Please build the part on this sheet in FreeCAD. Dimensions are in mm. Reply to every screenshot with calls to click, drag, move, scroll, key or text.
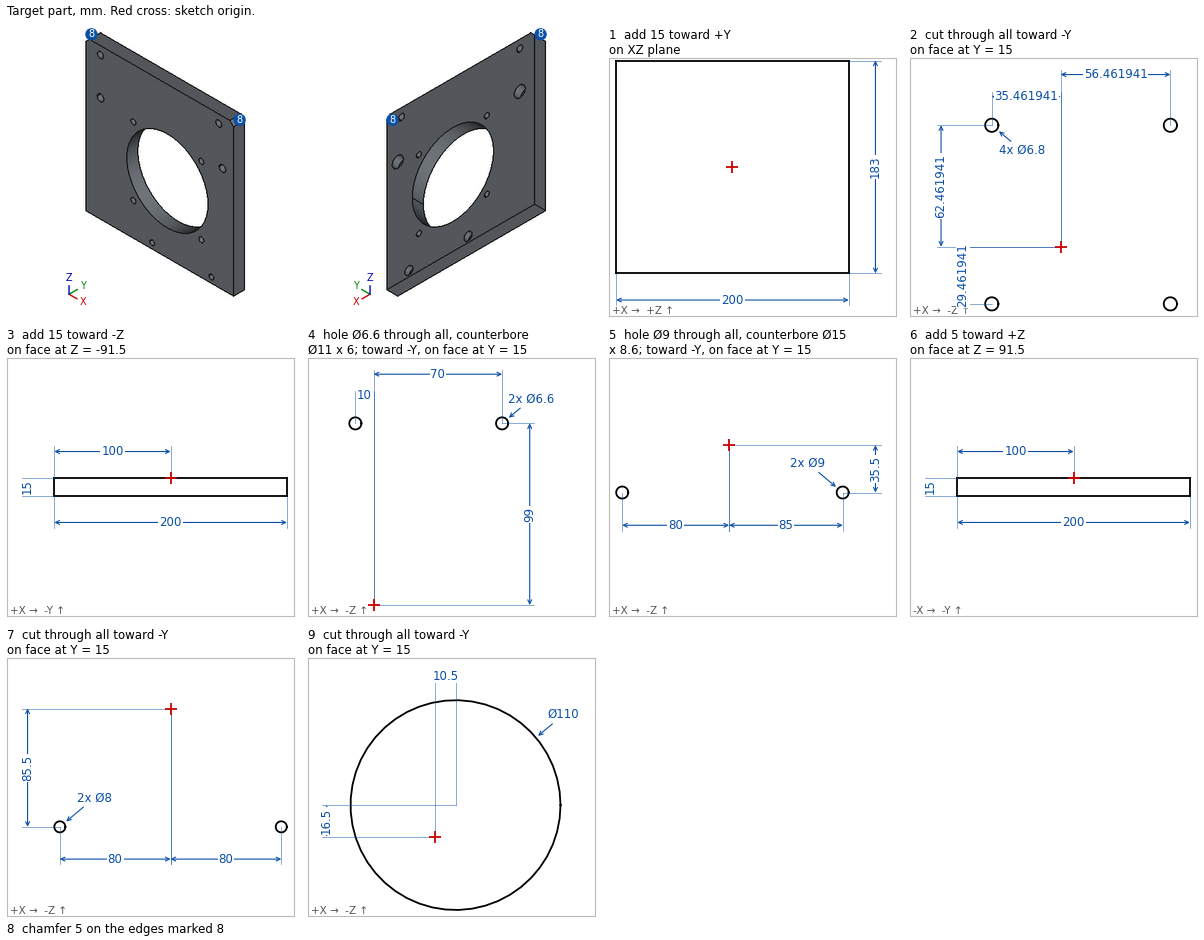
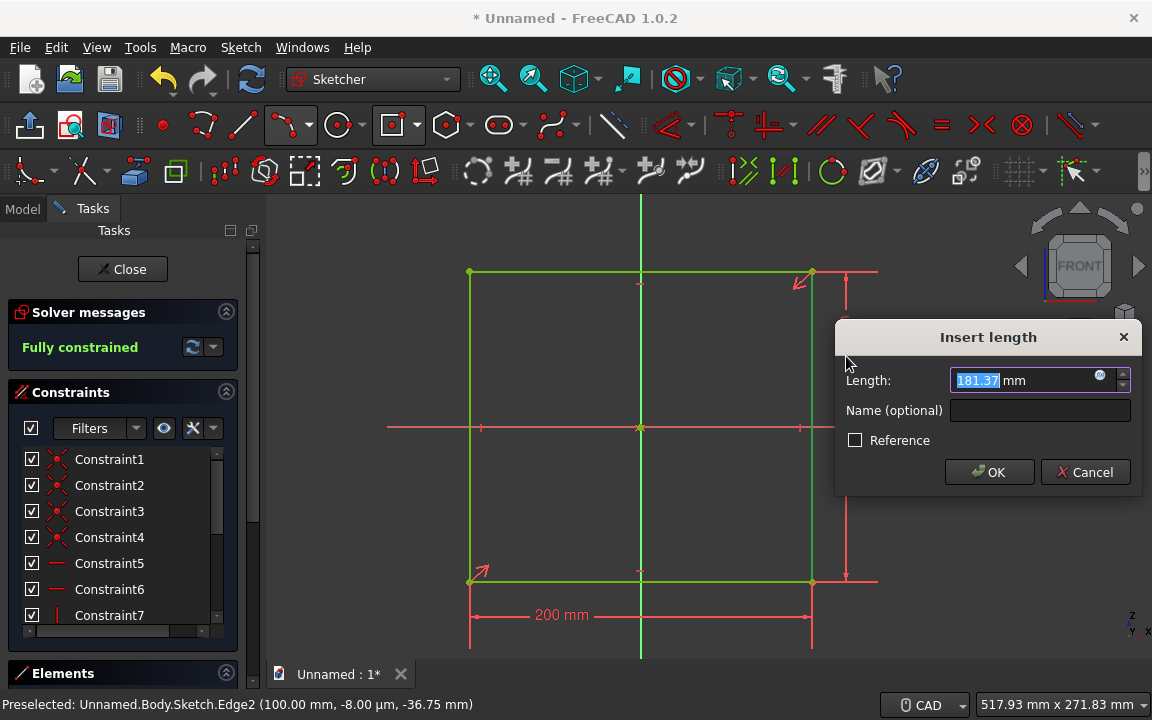
text(183)
key(Return)
key(Escape)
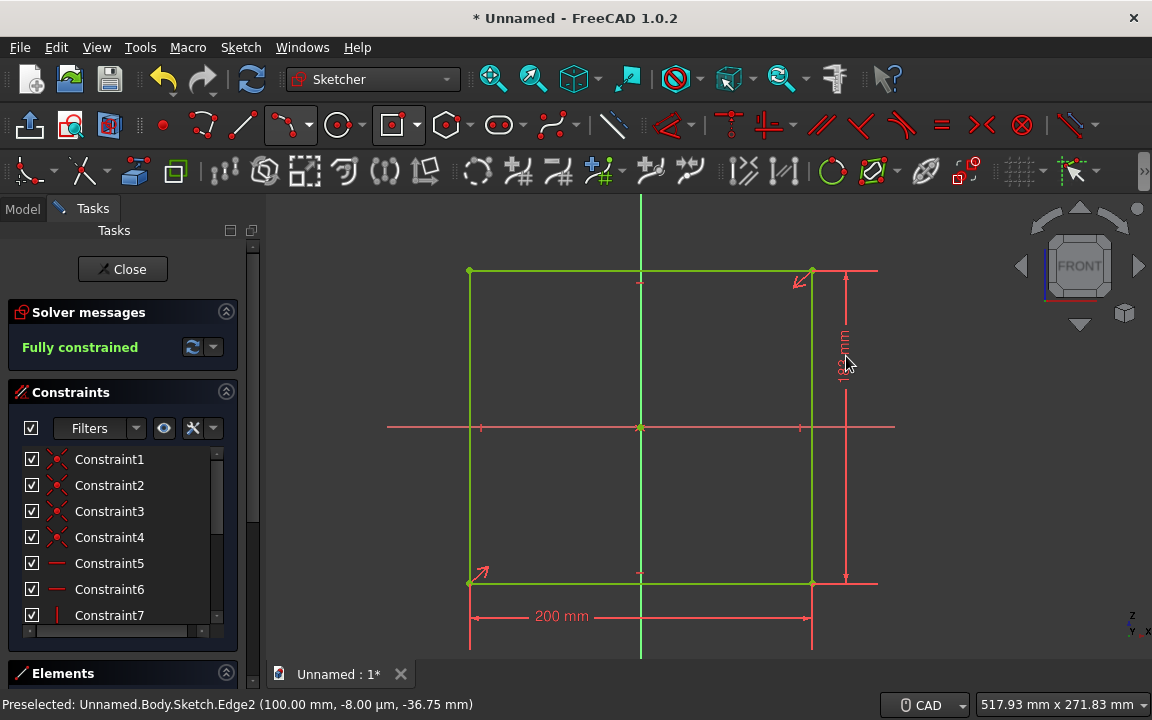
click(123, 269)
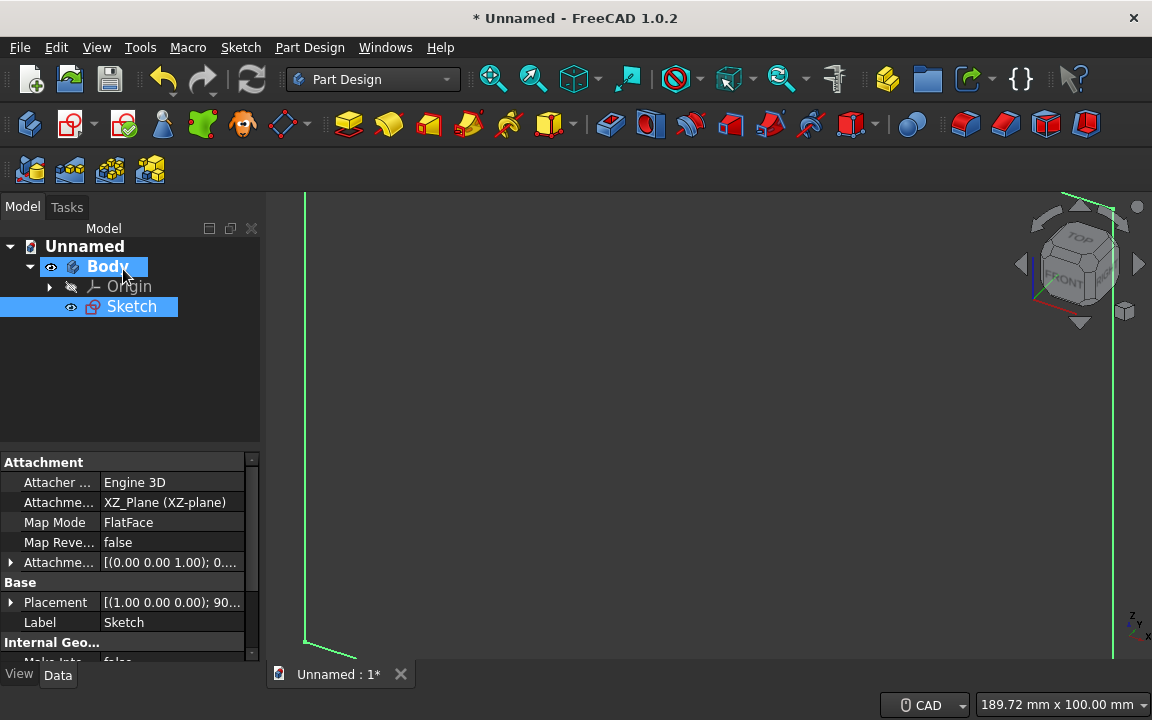
click(350, 124)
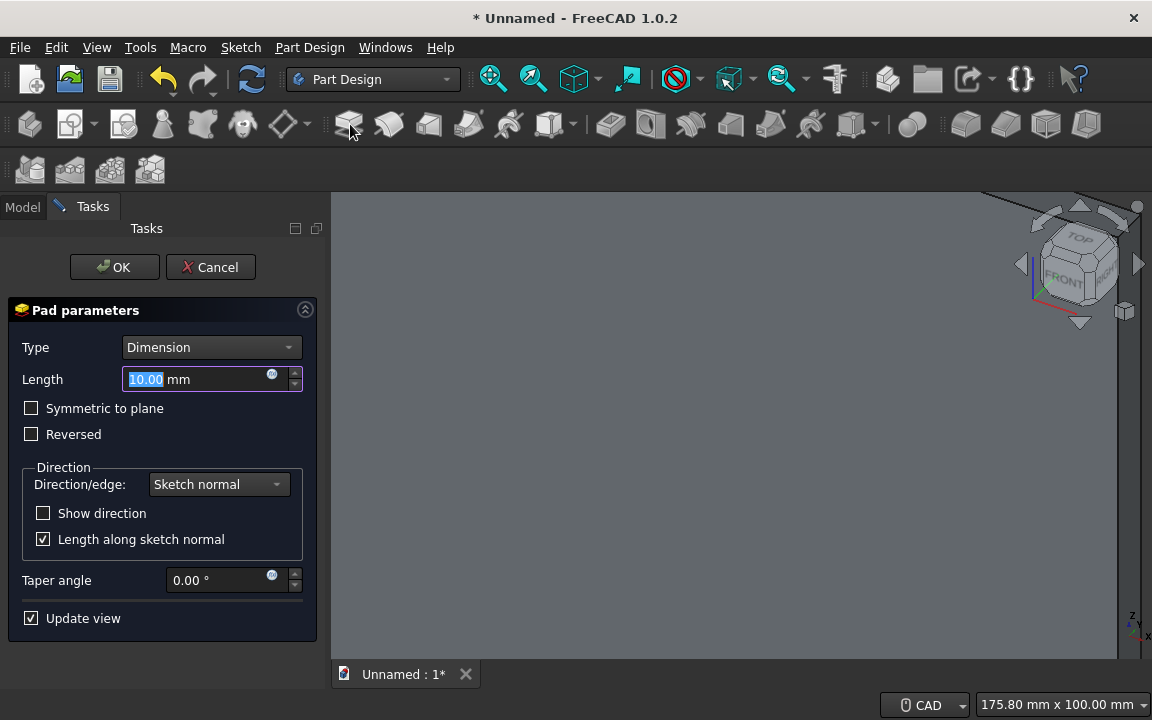
text(15)
key(Tab)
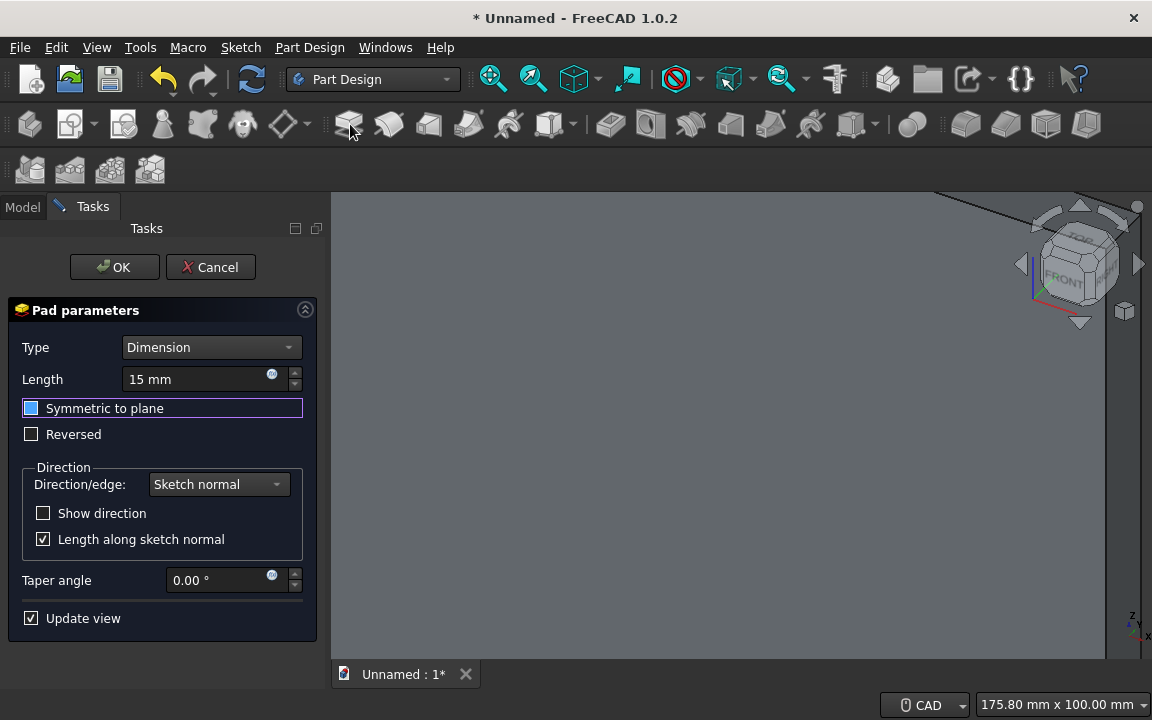
click(30, 434)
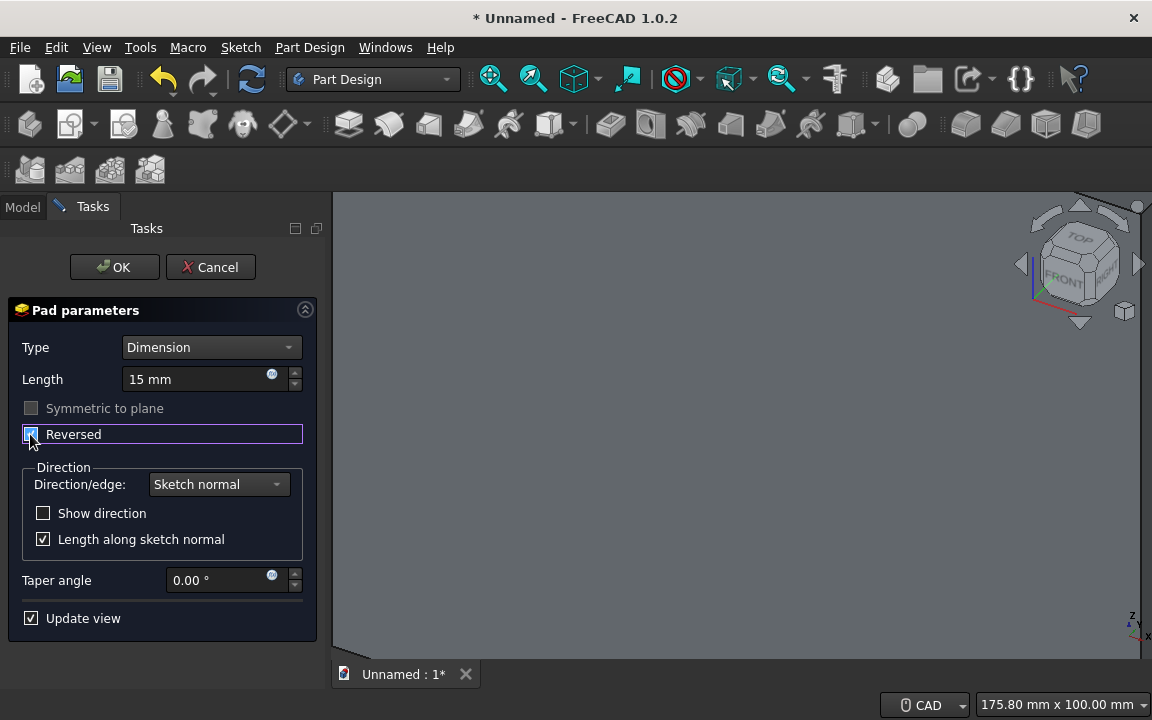
click(115, 267)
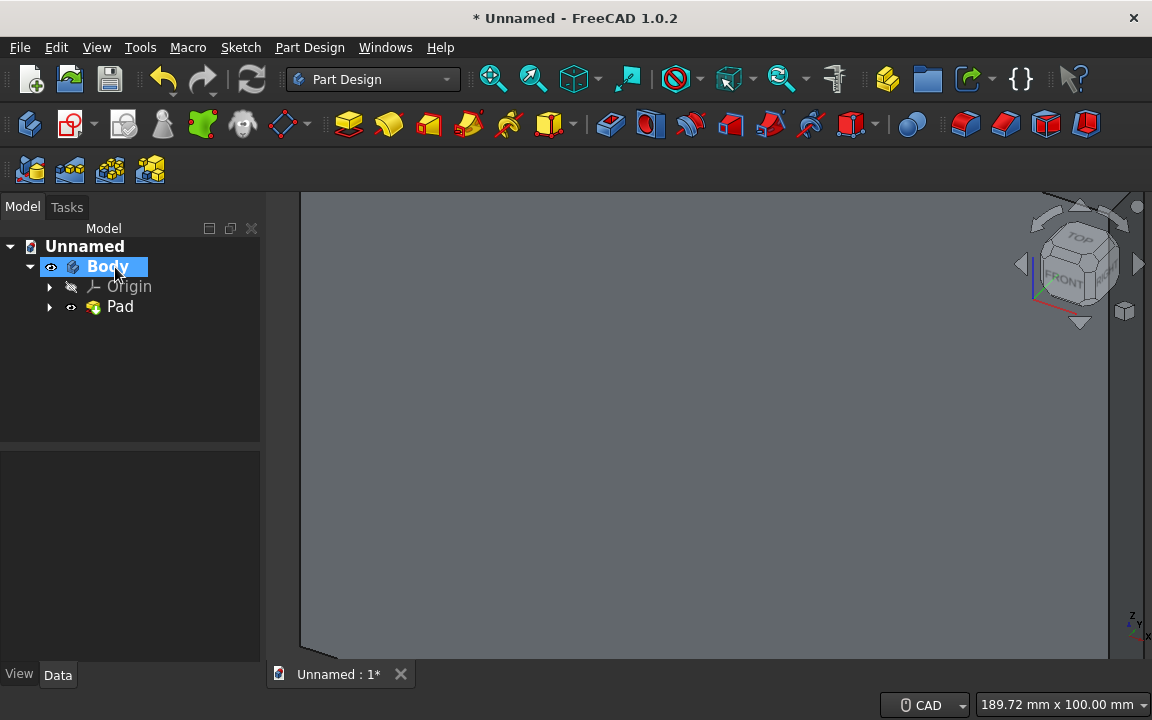
key(v)
key(f)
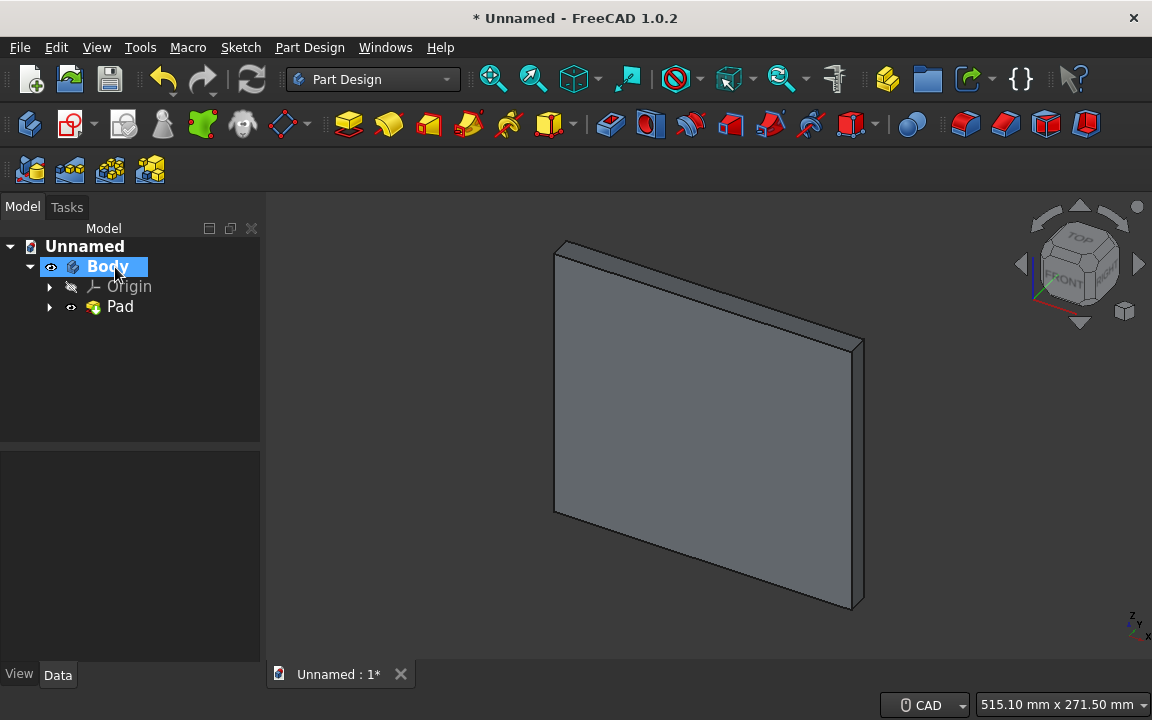
key(4)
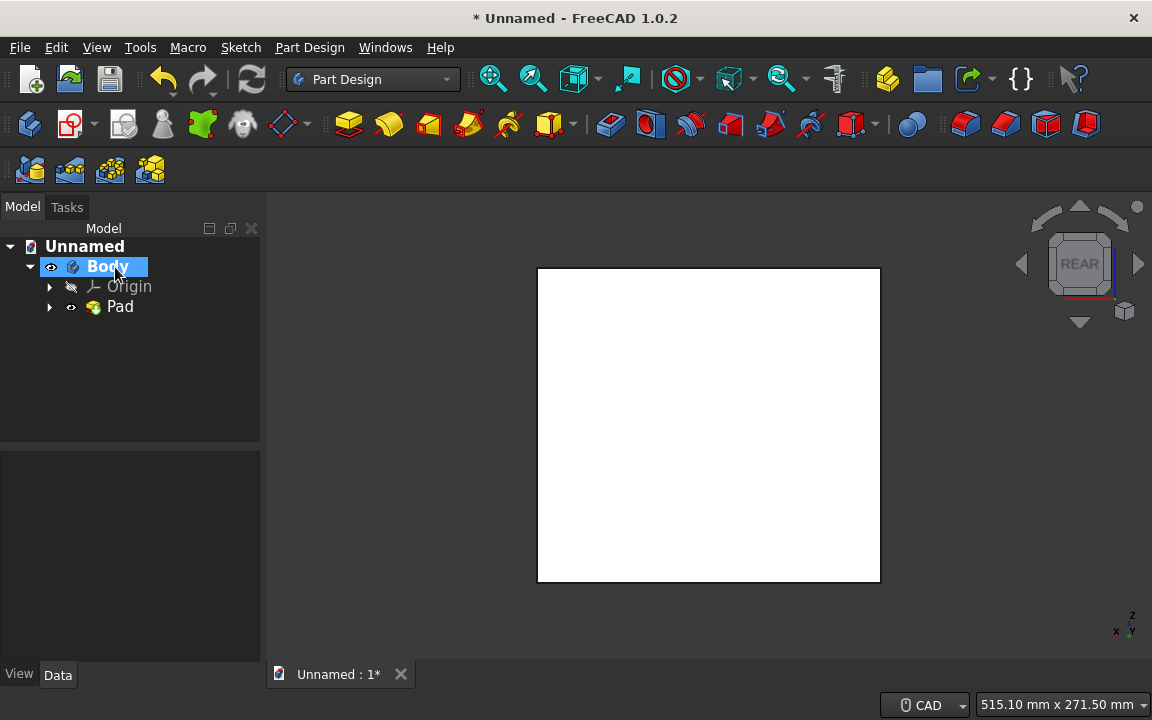
click(709, 424)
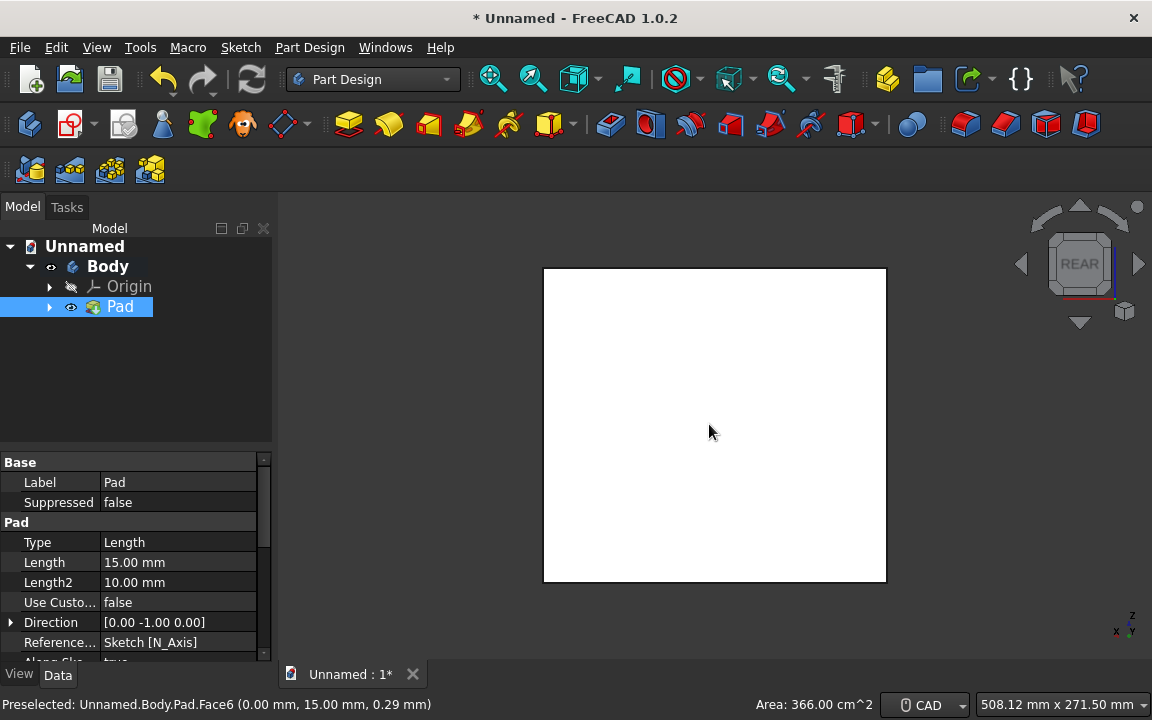
click(70, 124)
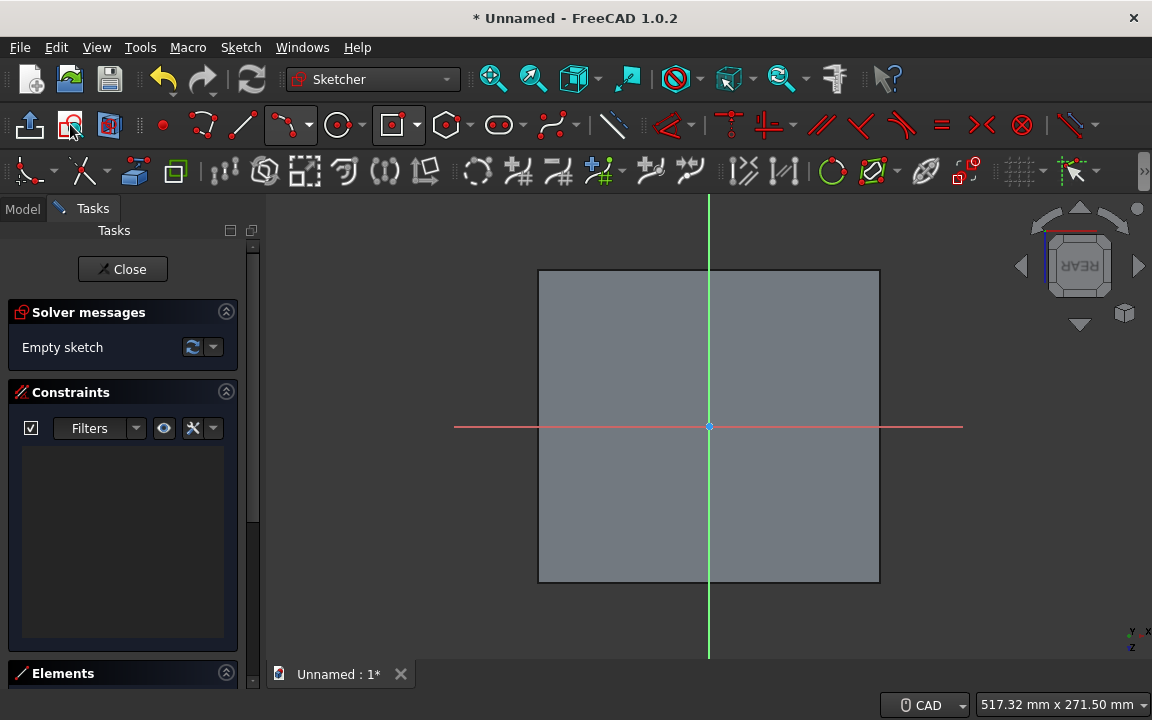
scroll(832, 364, up, 3)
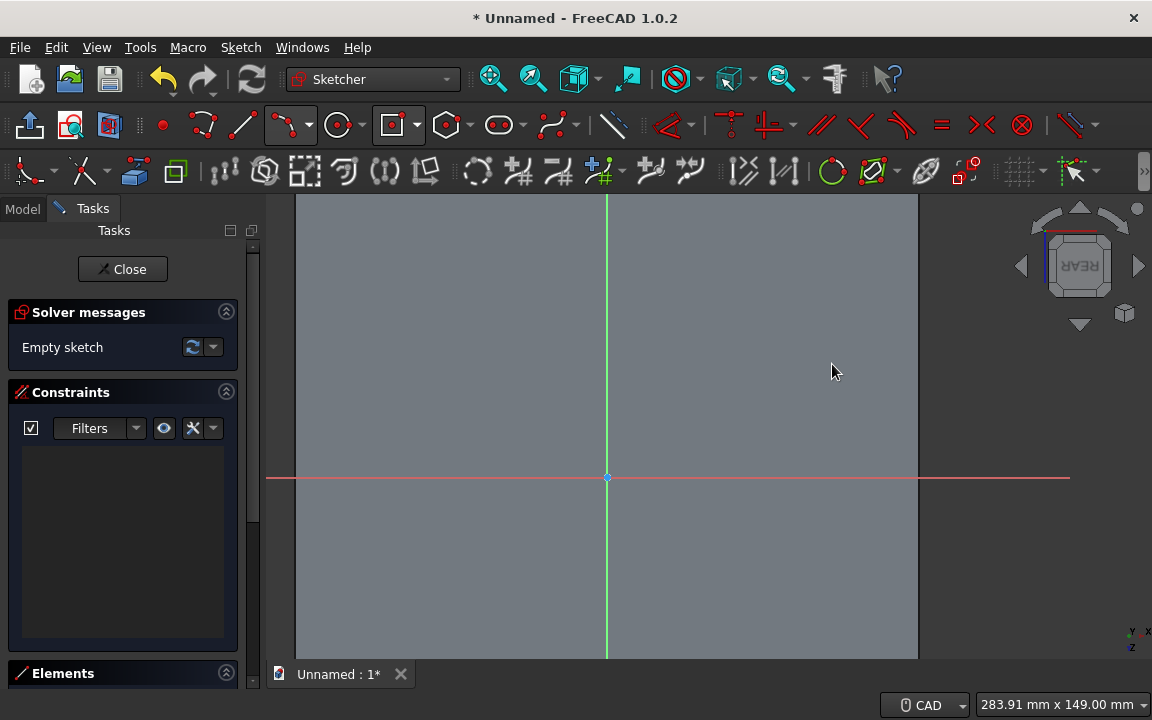
key(g)
key(c)